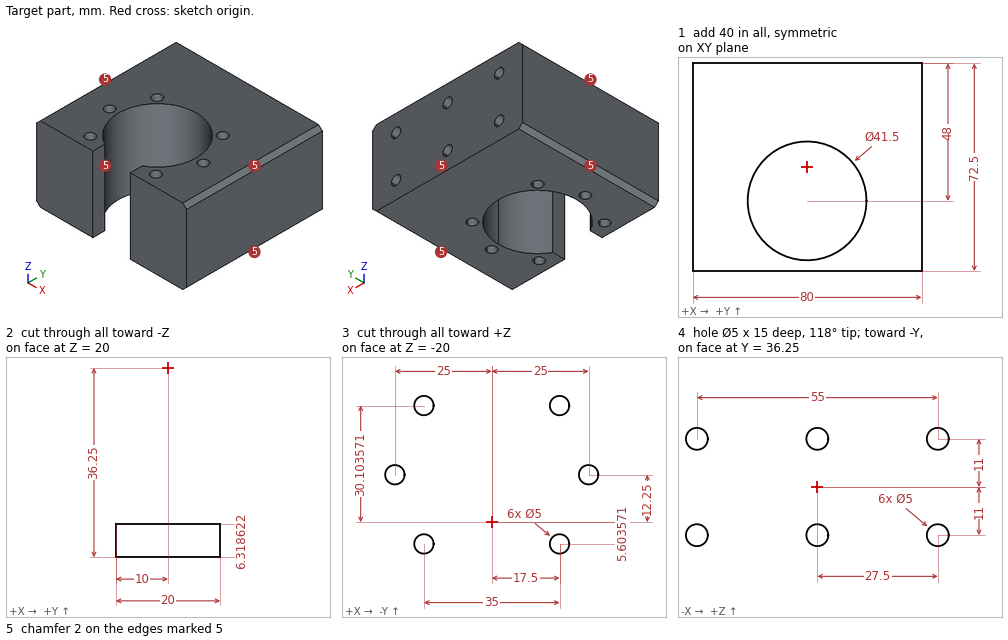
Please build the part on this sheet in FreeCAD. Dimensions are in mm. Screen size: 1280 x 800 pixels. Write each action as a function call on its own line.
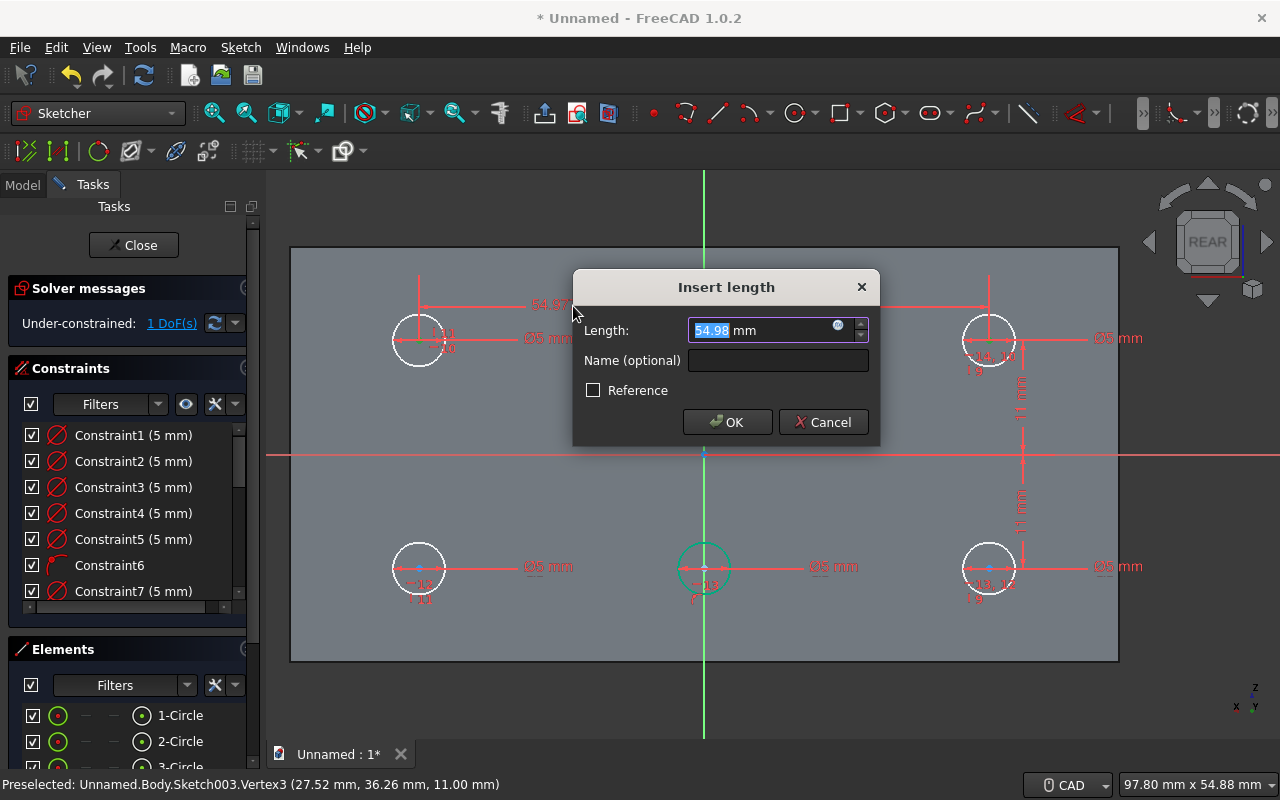
text(55)
key(Return)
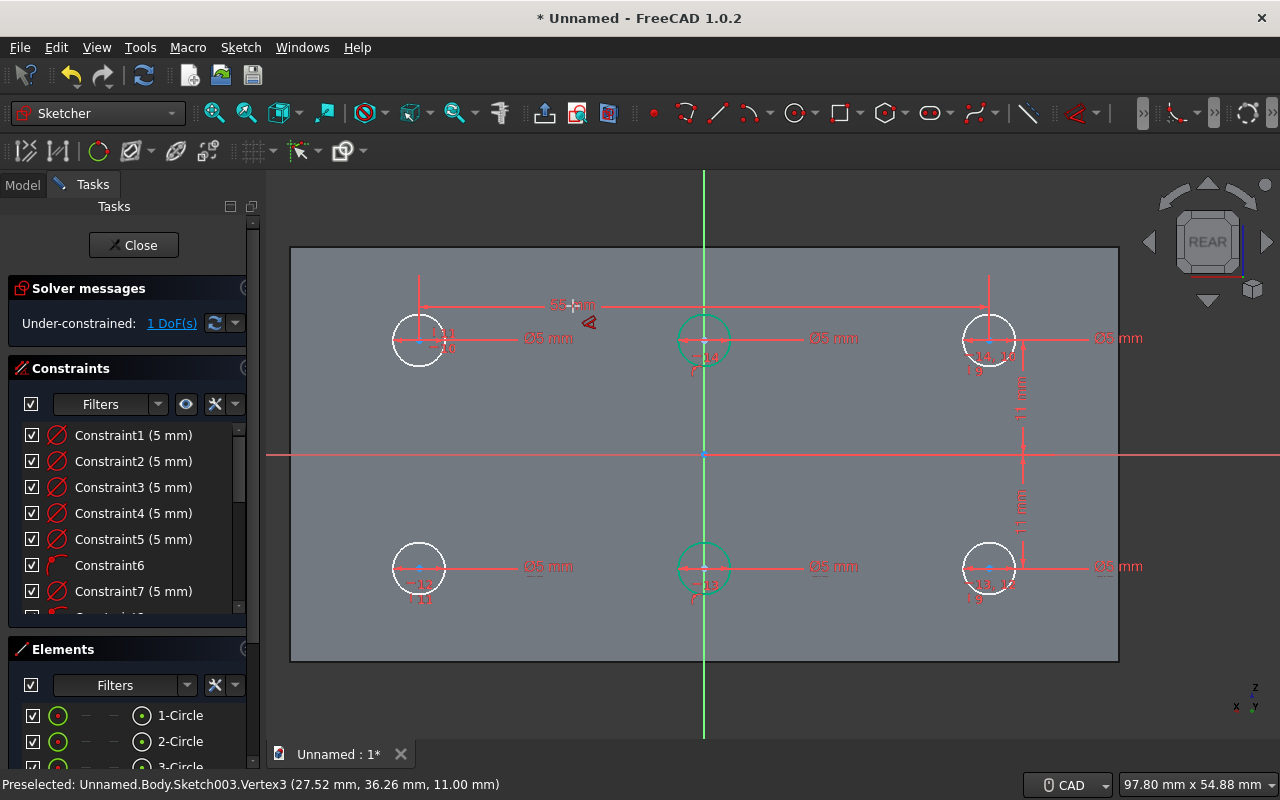
click(989, 569)
click(847, 603)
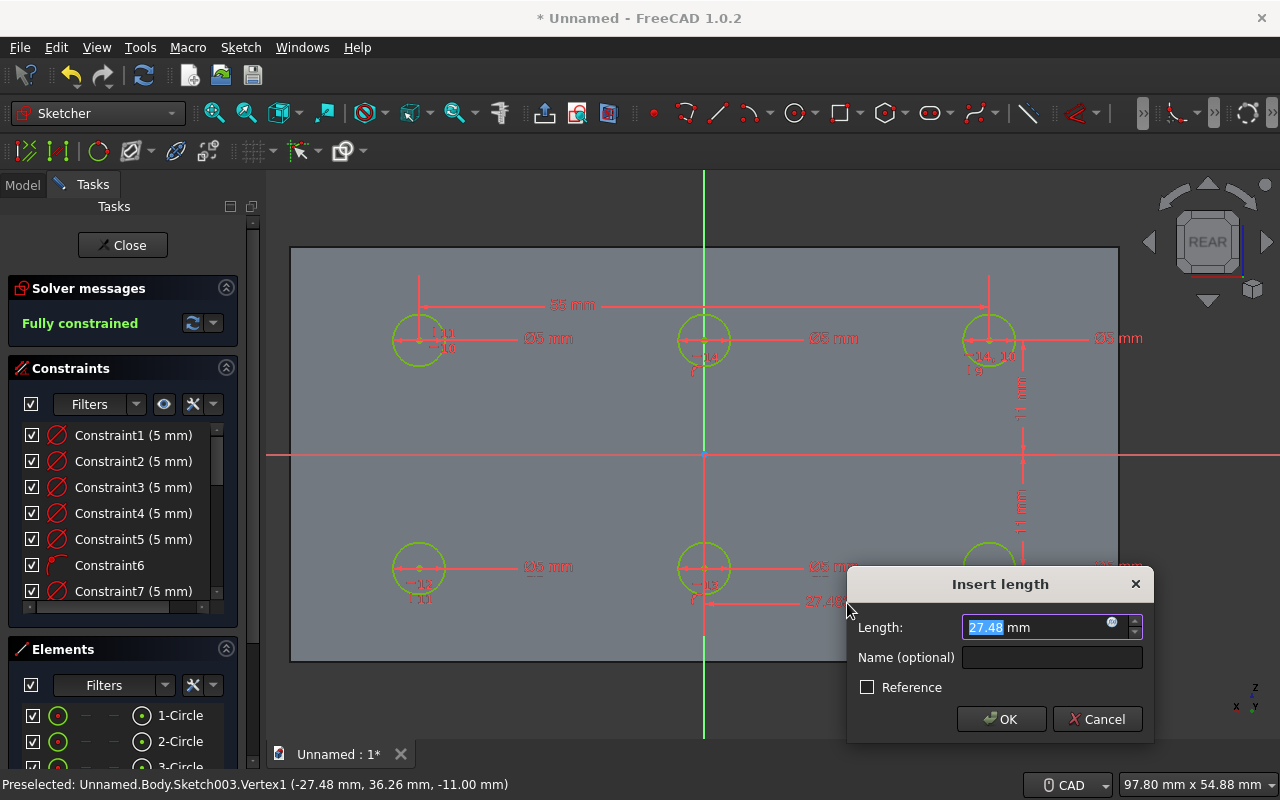
text(27.5)
key(Return)
key(Escape)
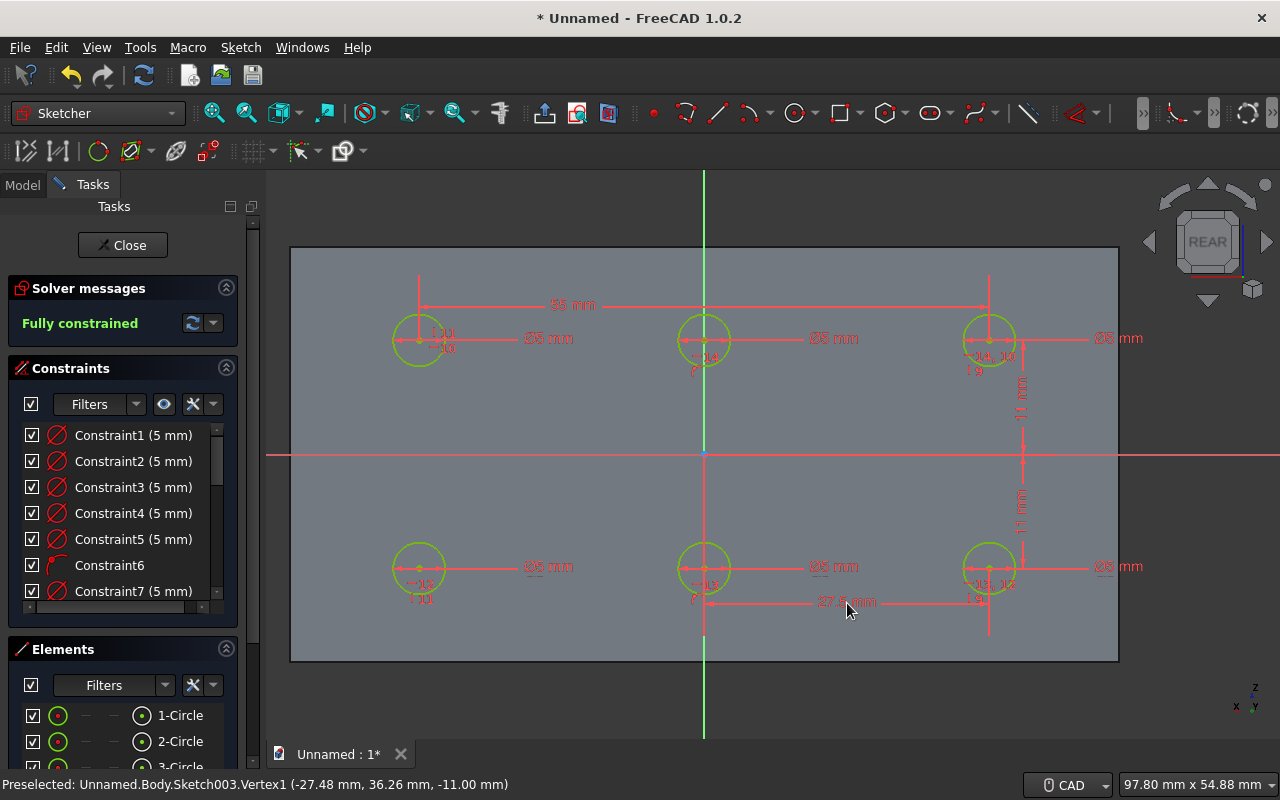
click(123, 245)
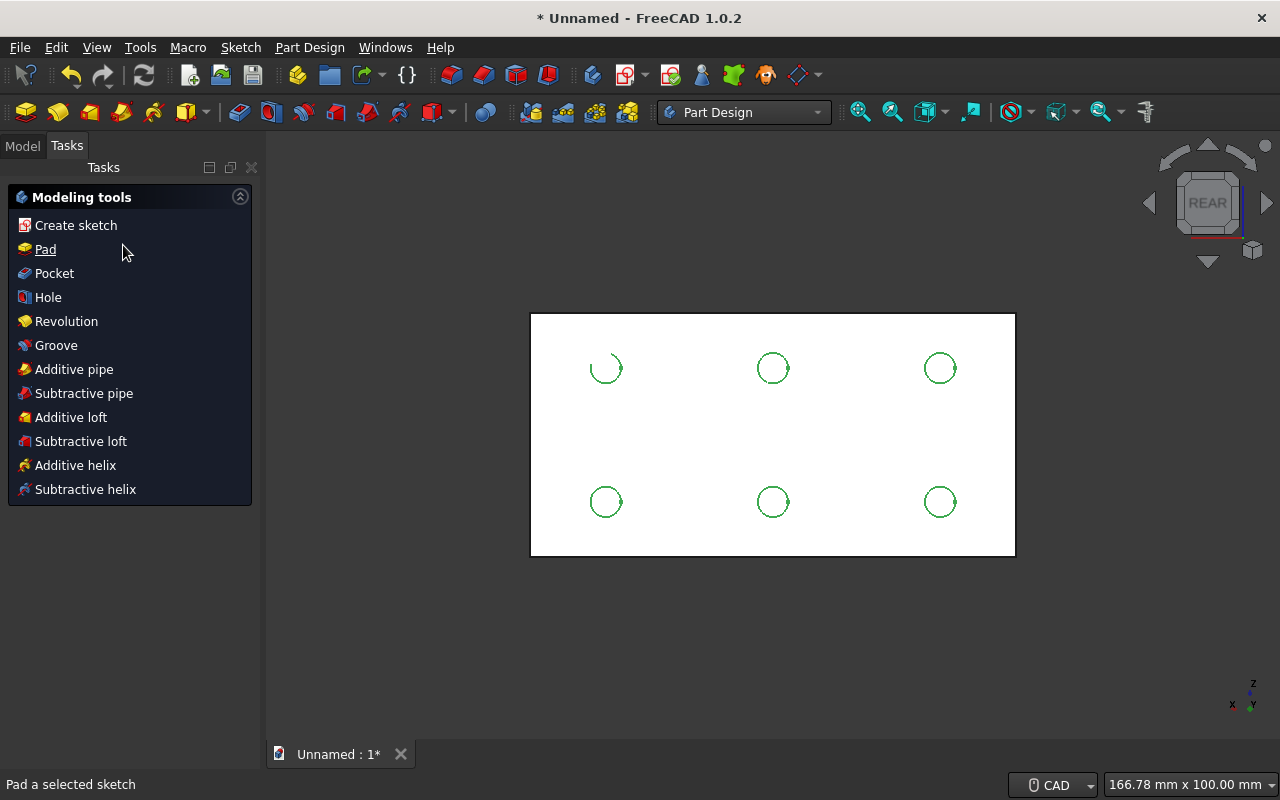
click(272, 112)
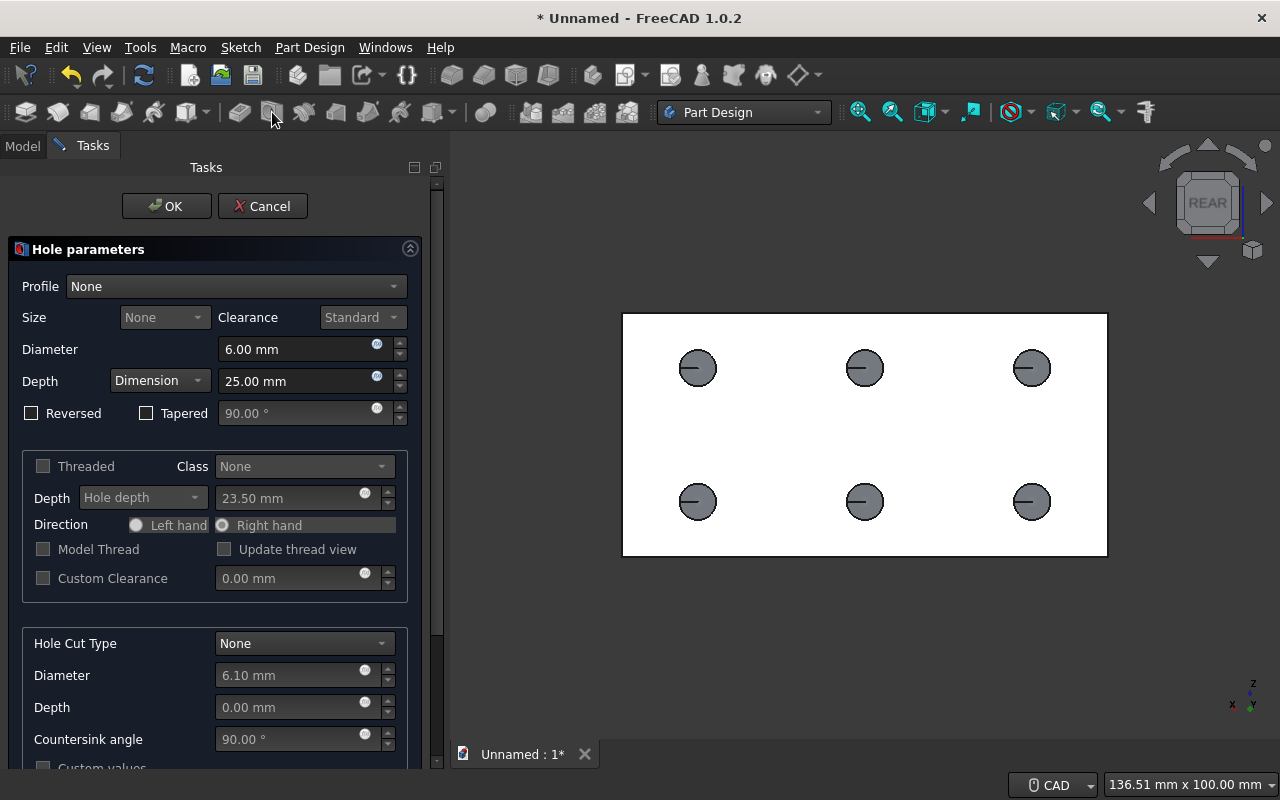
triple_click(305, 349)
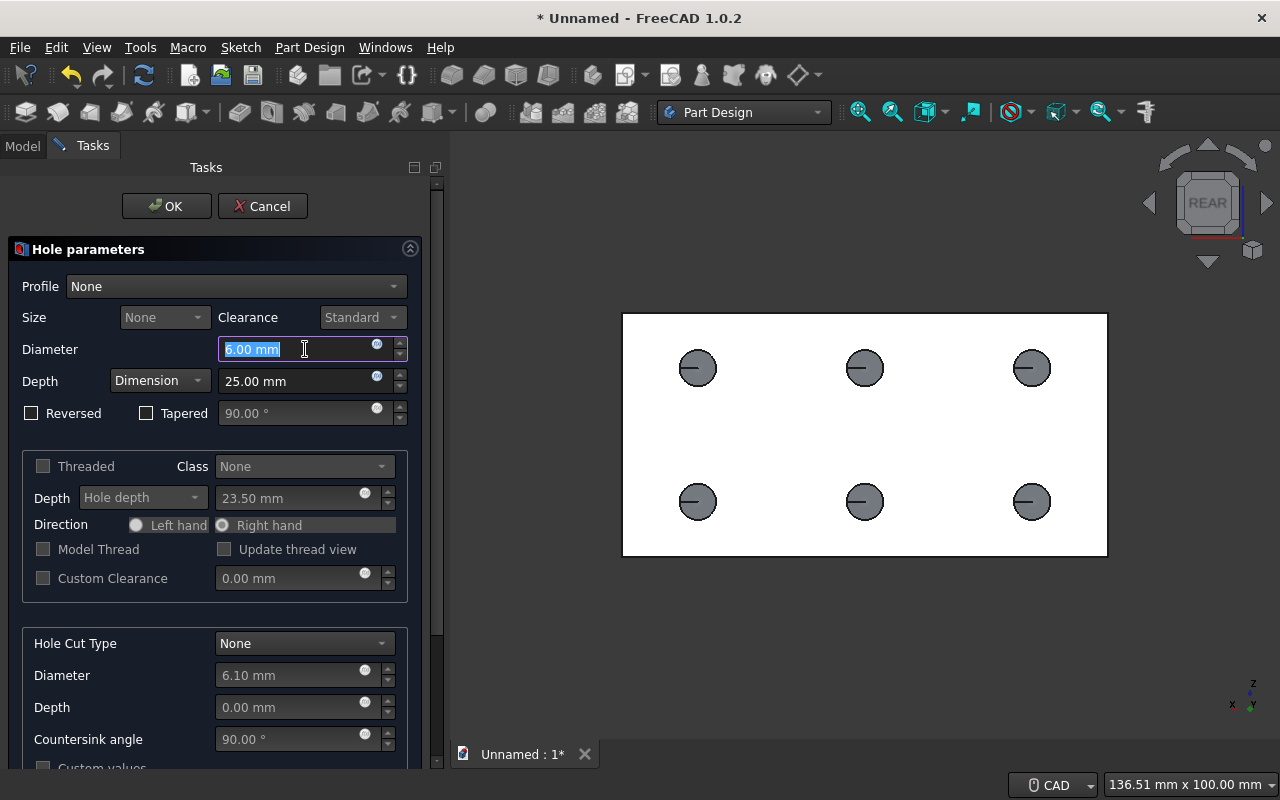
text(5)
key(Tab)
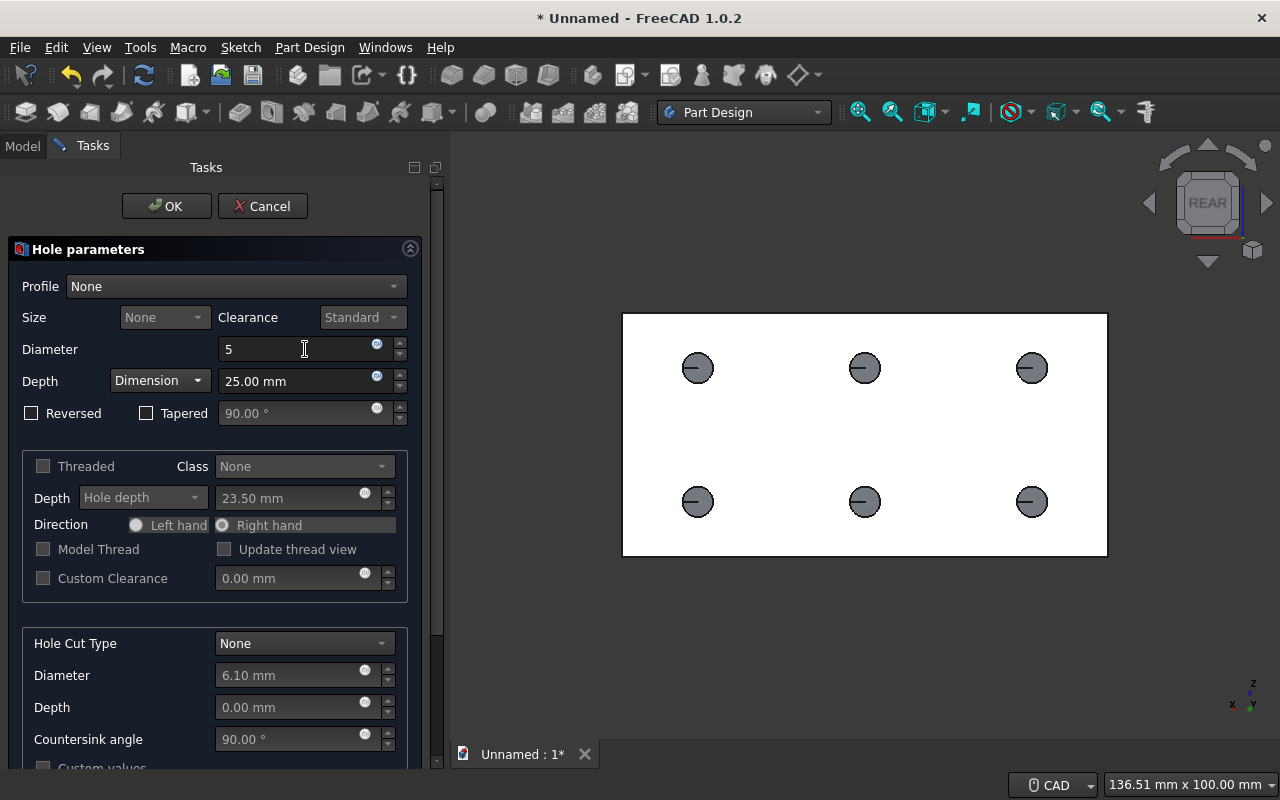
triple_click(305, 381)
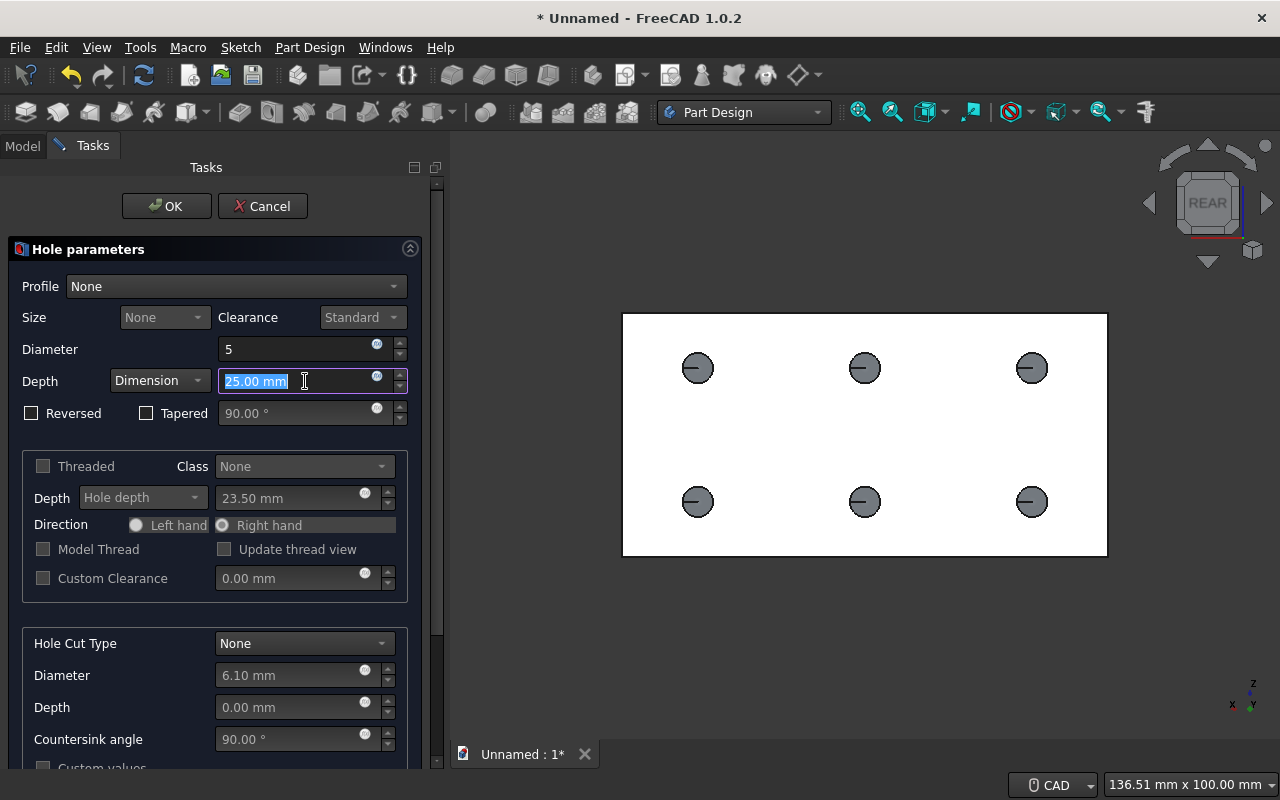
text(15)
key(Tab)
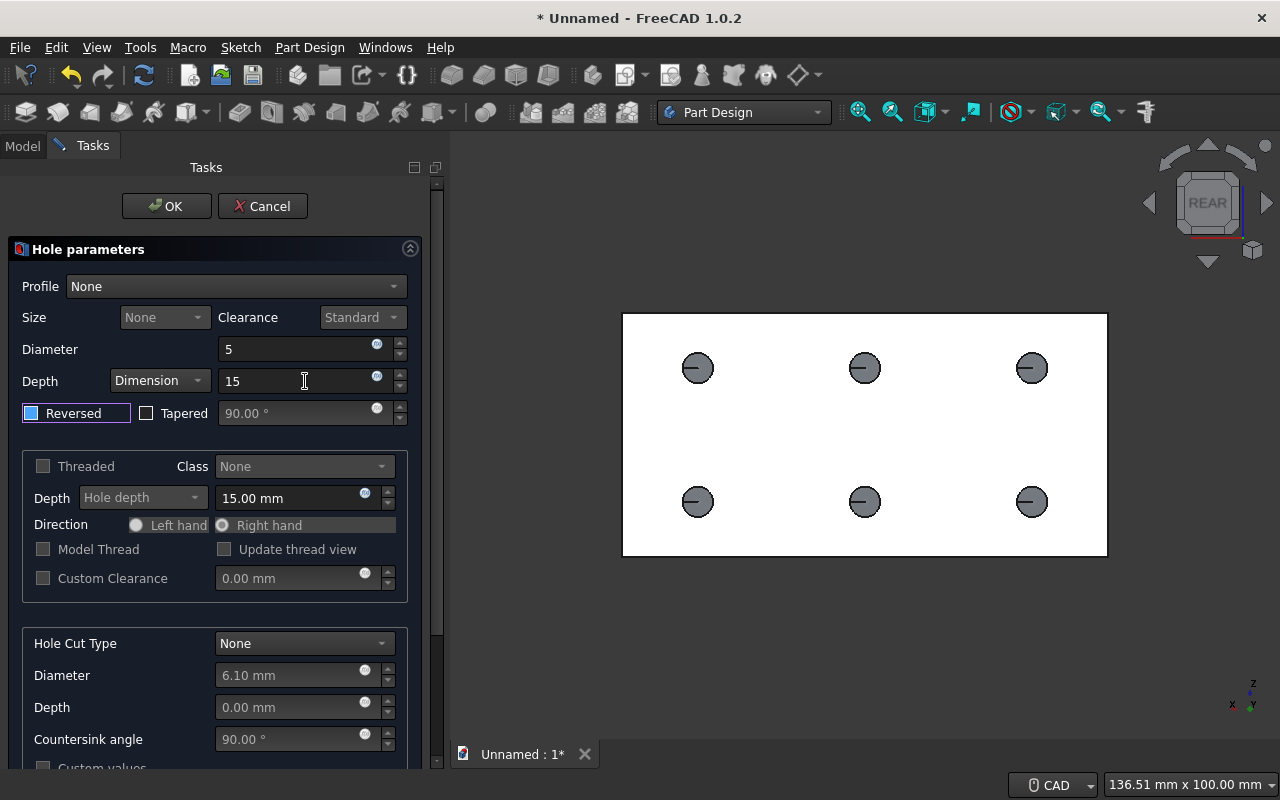
click(167, 206)